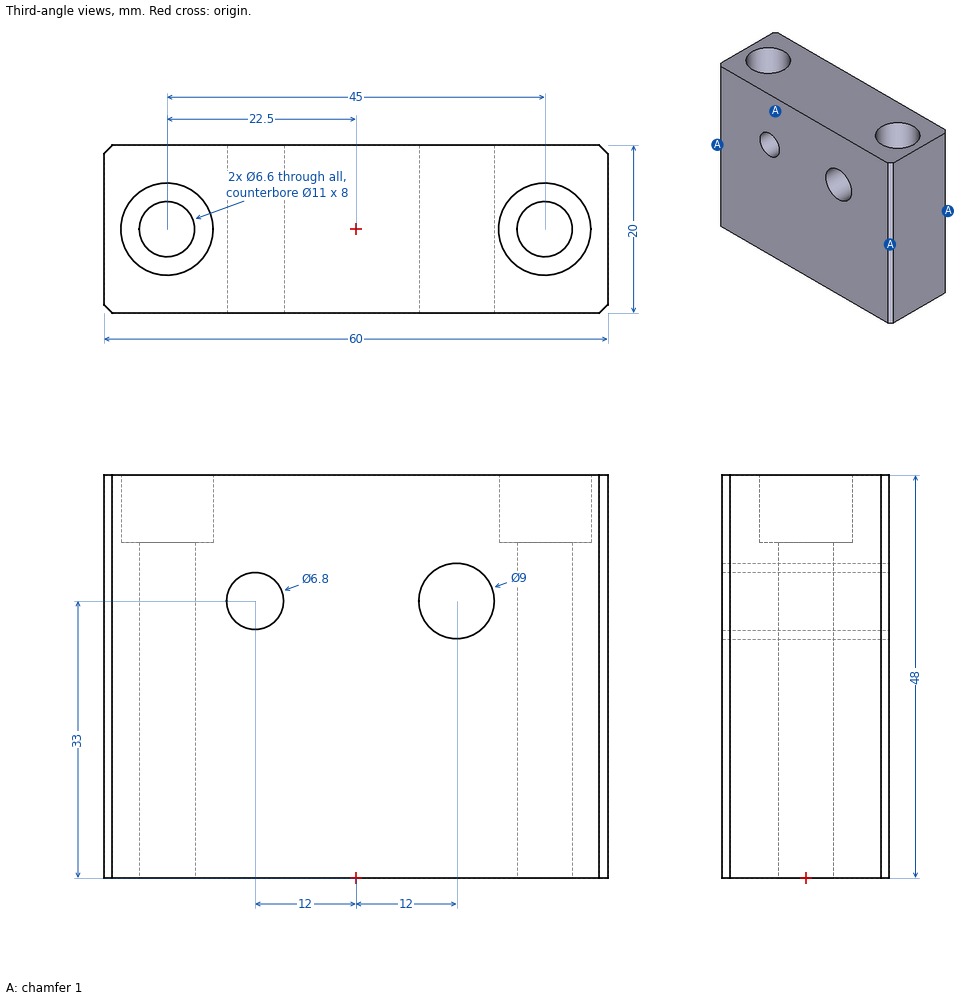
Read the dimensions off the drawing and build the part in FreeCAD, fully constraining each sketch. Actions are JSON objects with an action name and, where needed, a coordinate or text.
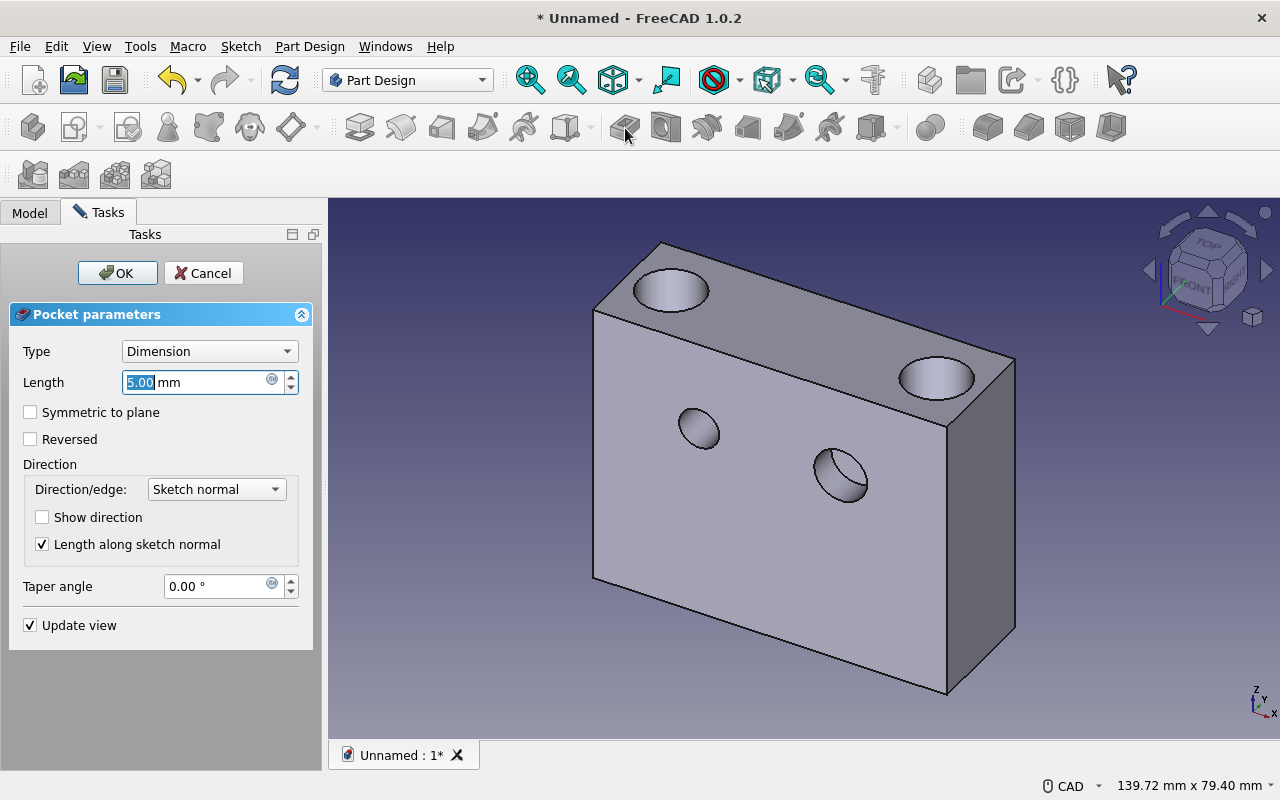
{"action": "left_click", "coordinate": [210, 352]}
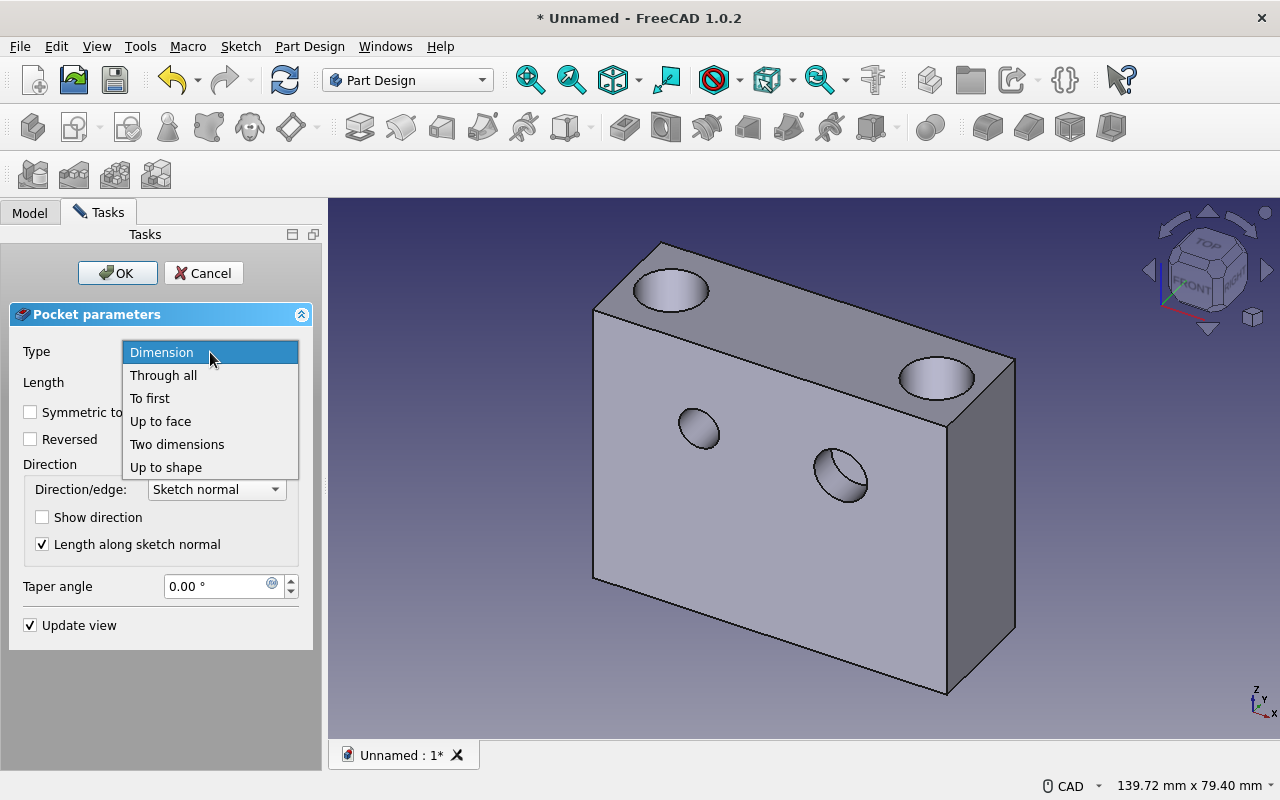
{"action": "left_click", "coordinate": [208, 376]}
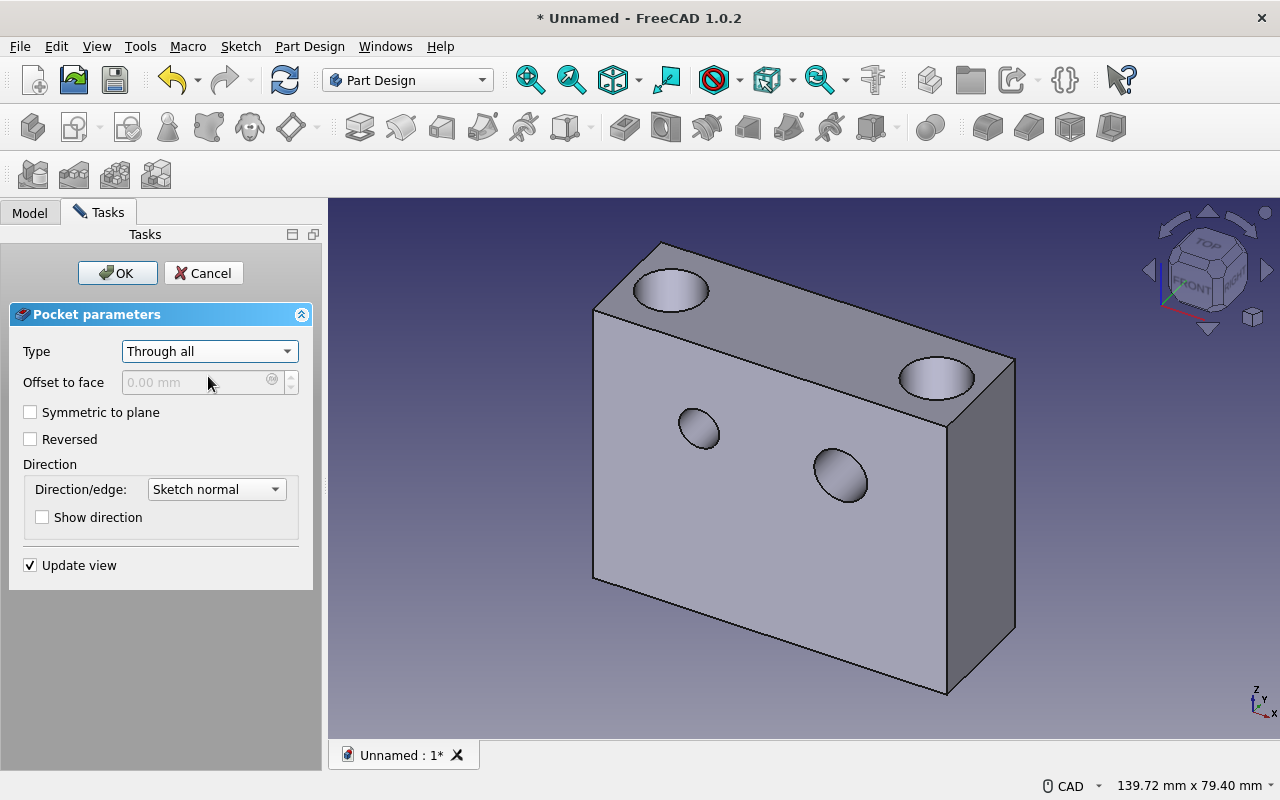
{"action": "left_click", "coordinate": [118, 273]}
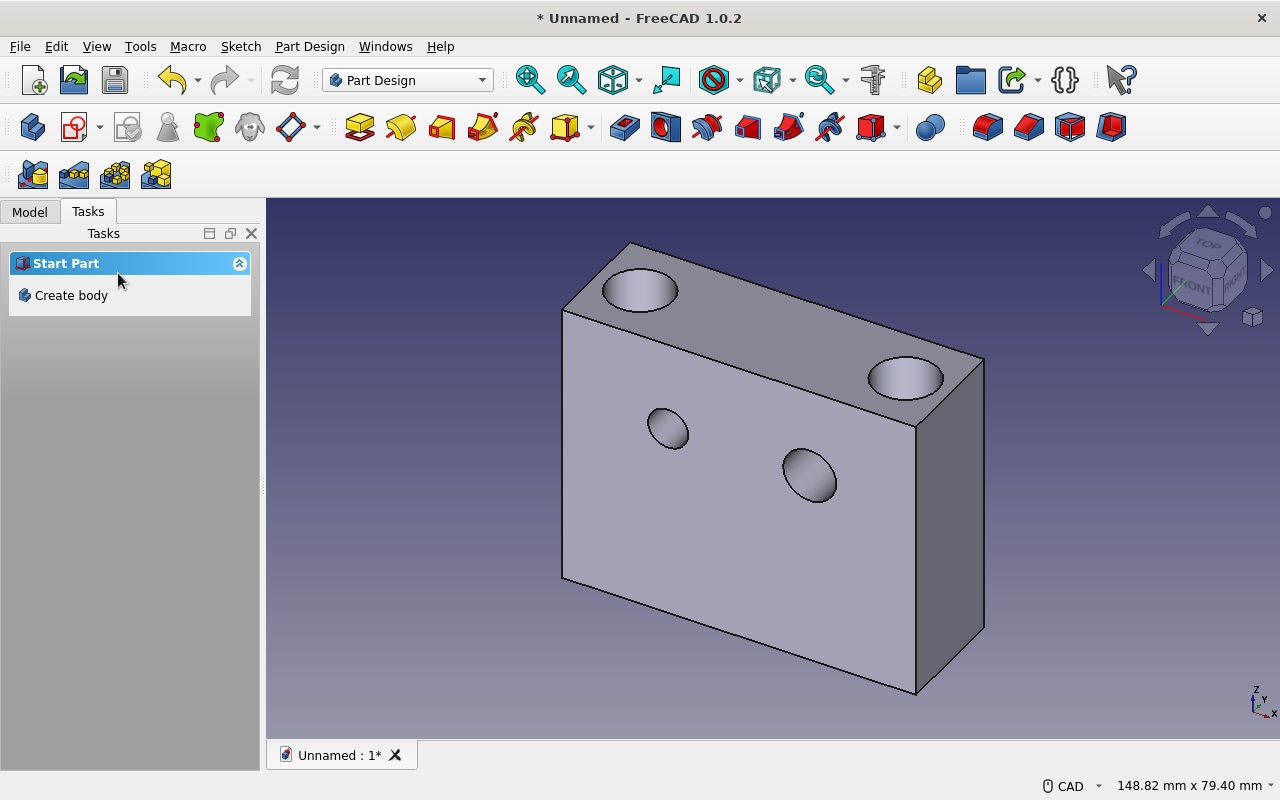
{"action": "left_click", "coordinate": [916, 560]}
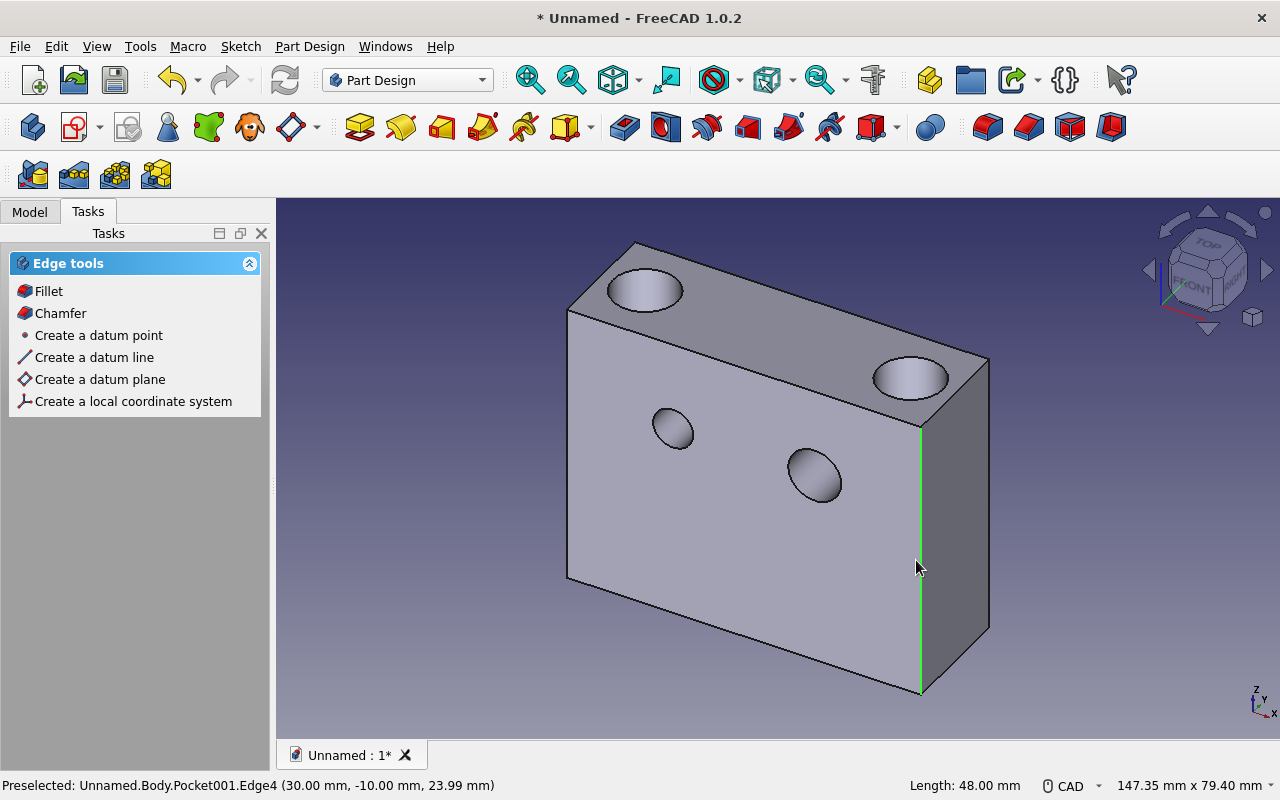
{"action": "key", "text": "0"}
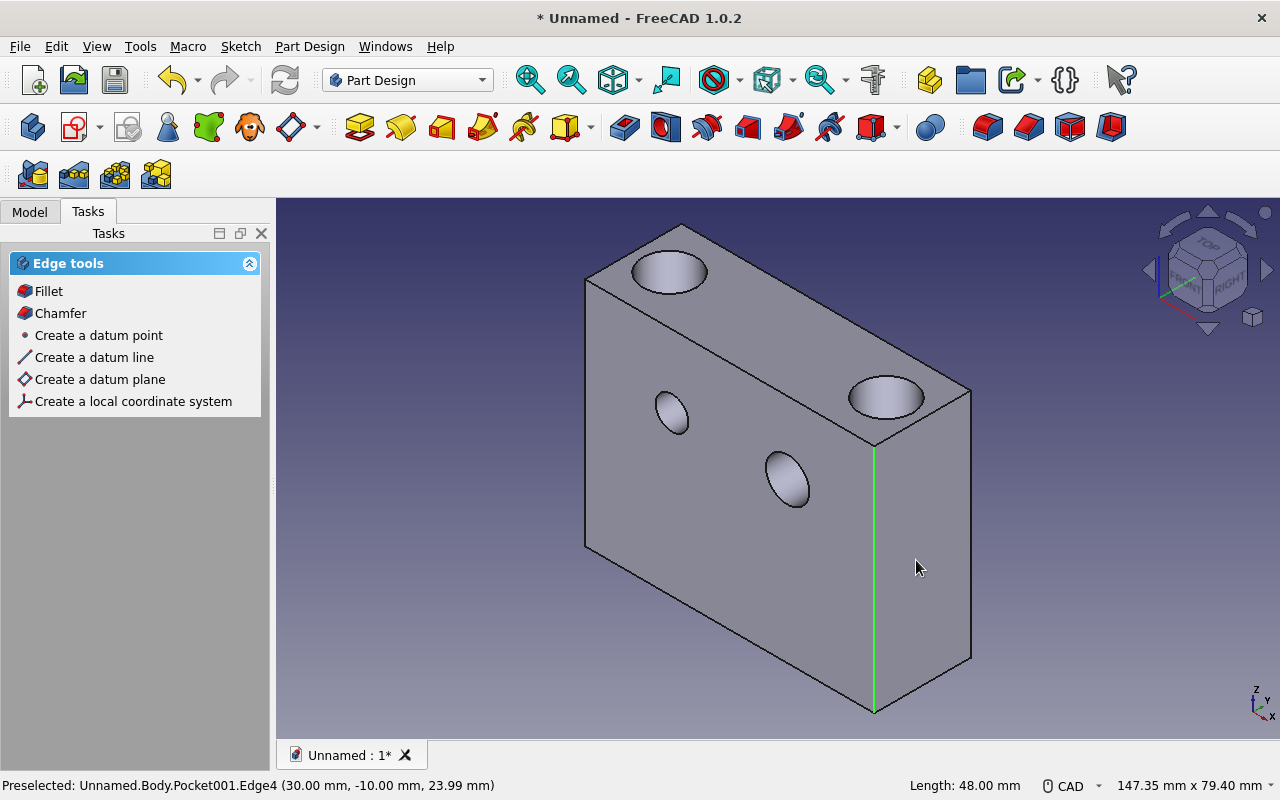
{"action": "key", "text": "2"}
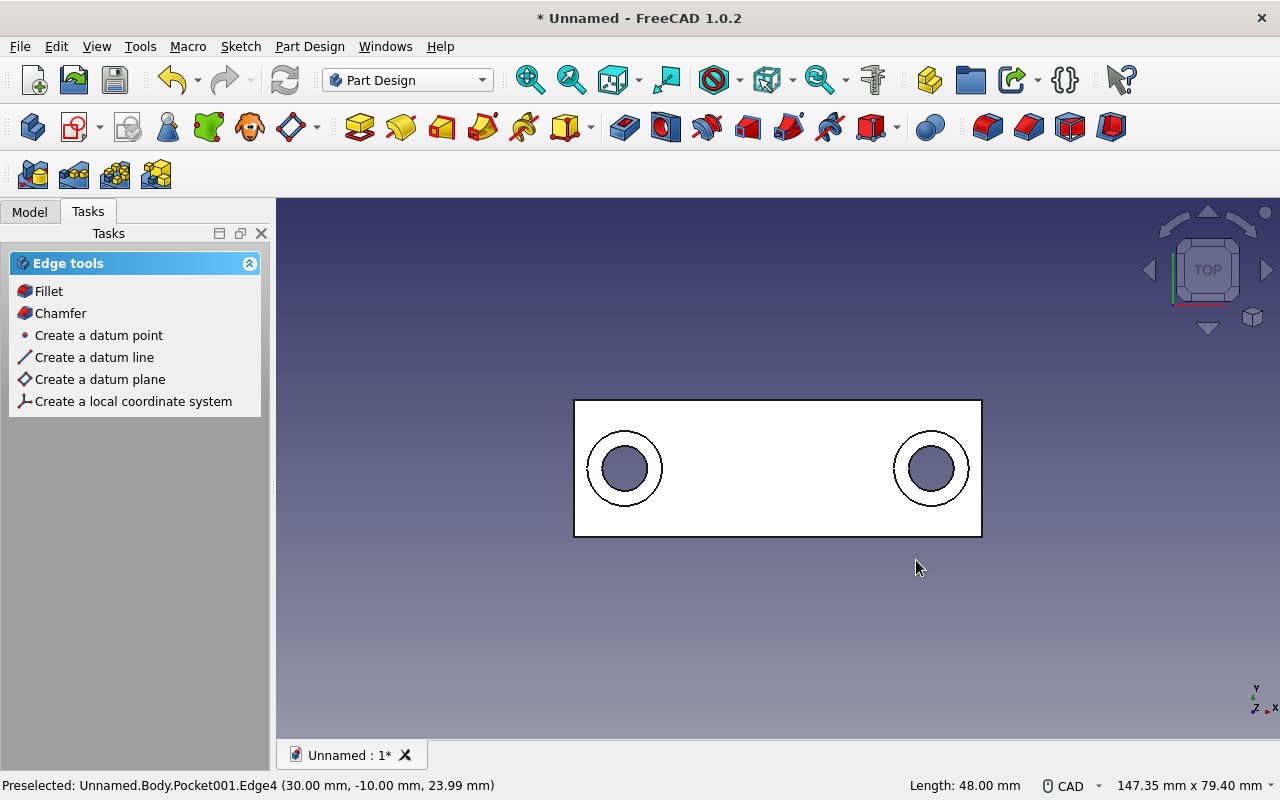
{"action": "left_click", "coordinate": [531, 80]}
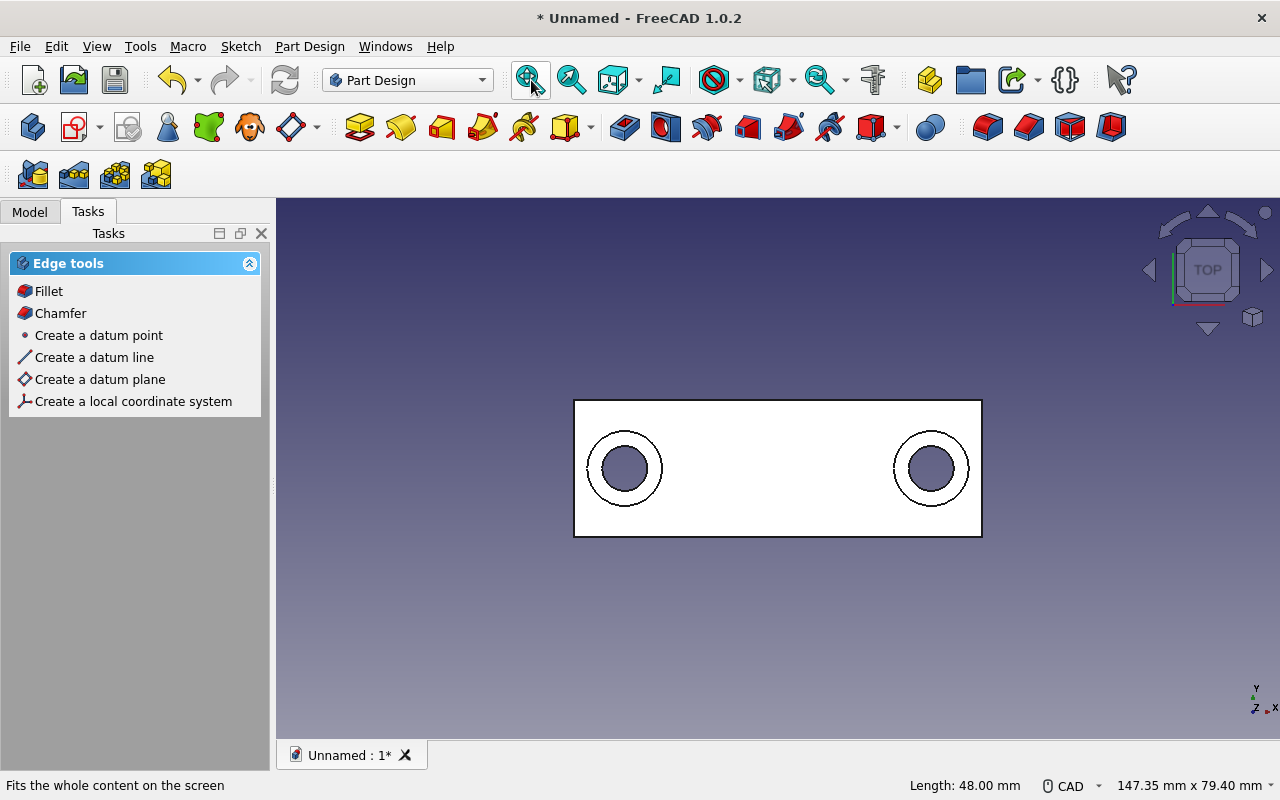
{"action": "key", "text": "1"}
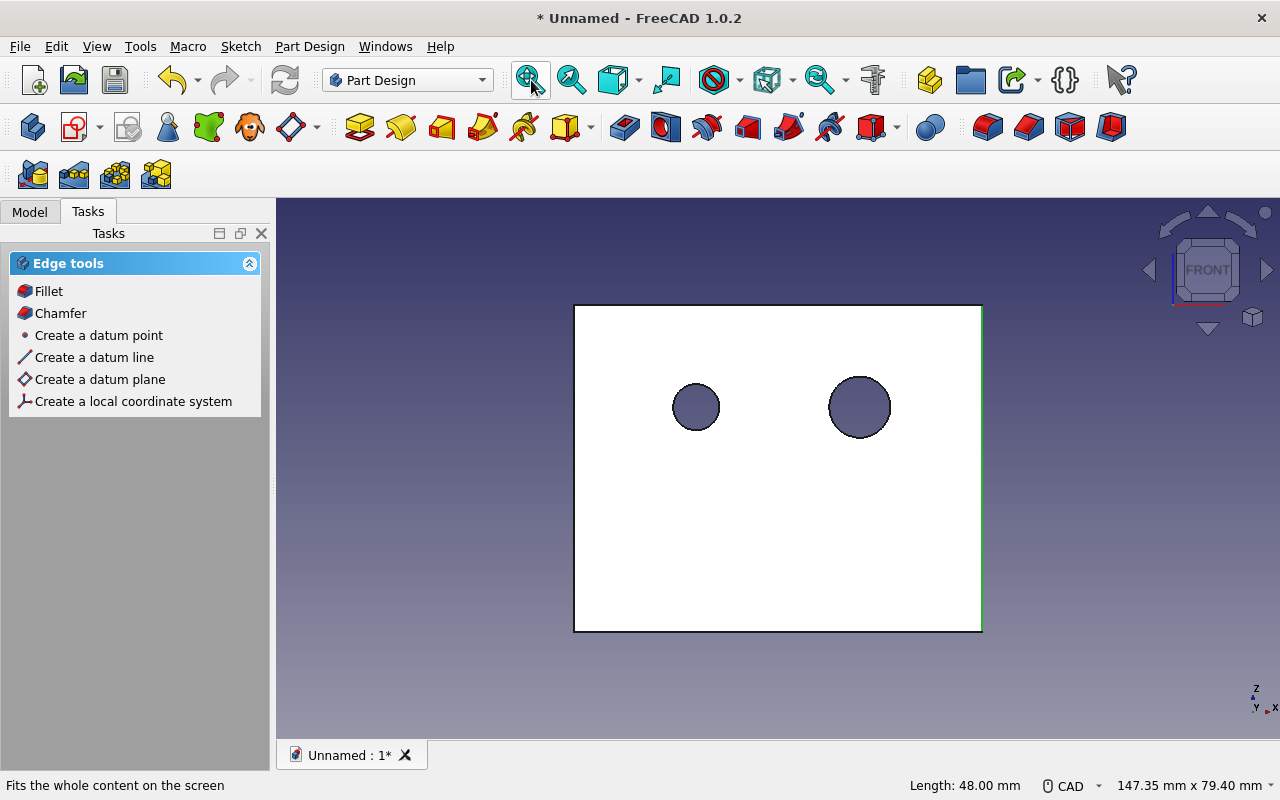
{"action": "left_click", "coordinate": [574, 467], "text": "ctrl"}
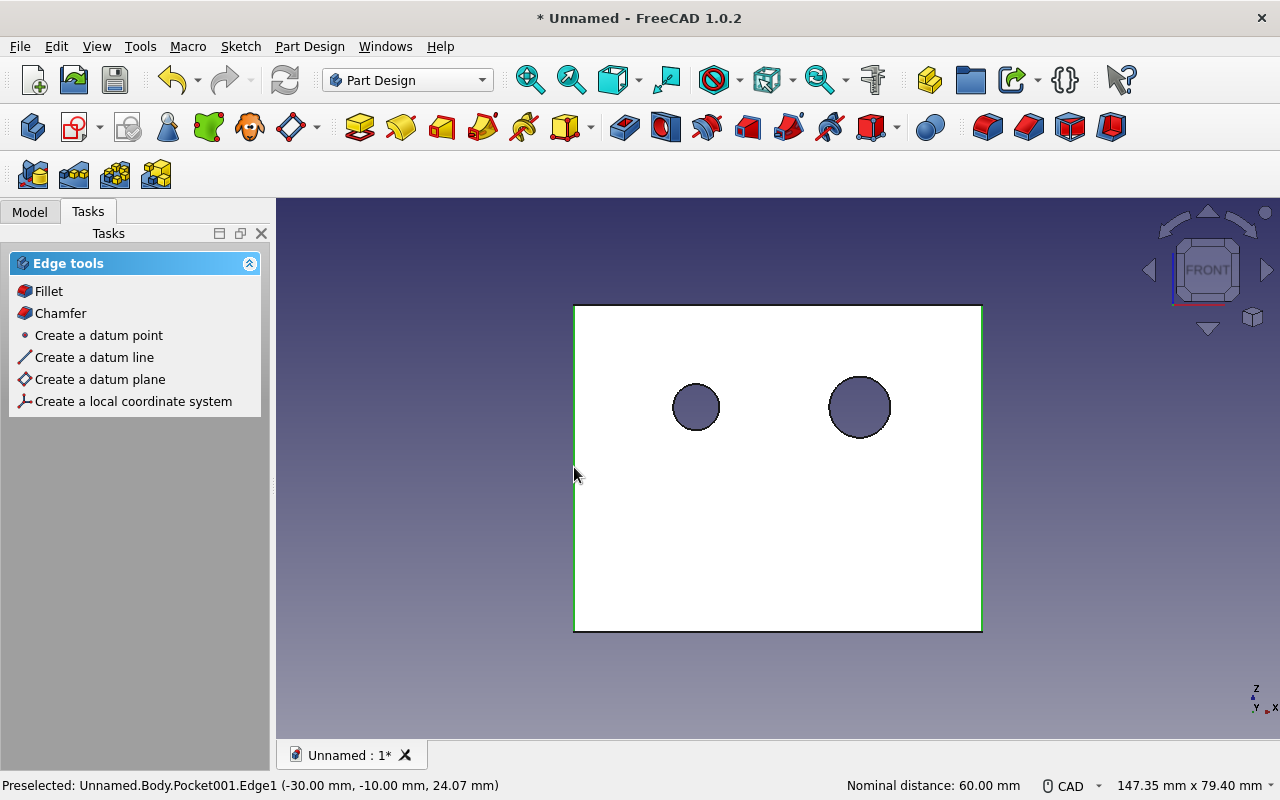
{"action": "key", "text": "3"}